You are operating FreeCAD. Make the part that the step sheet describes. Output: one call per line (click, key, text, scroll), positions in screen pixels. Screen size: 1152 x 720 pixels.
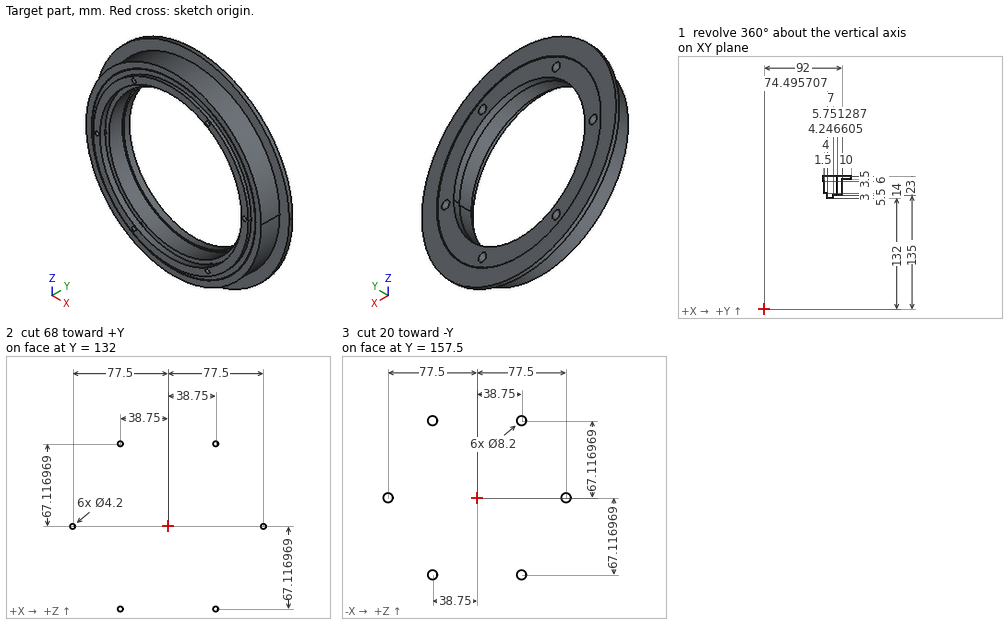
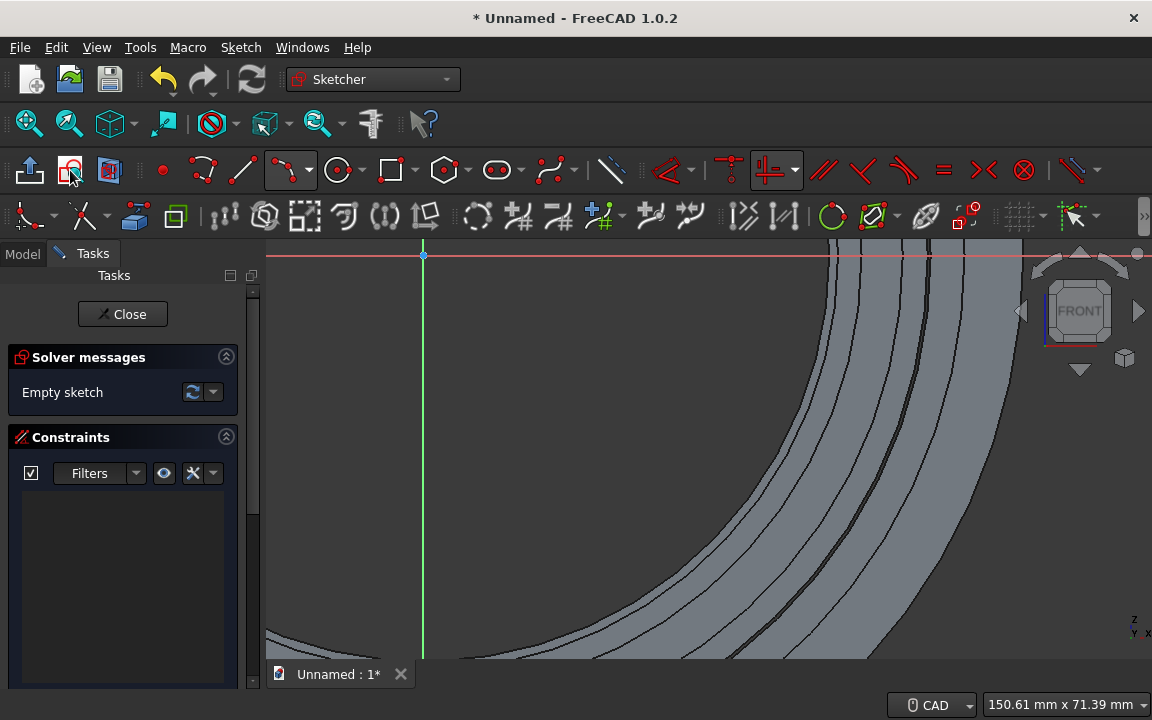
scroll(734, 532, down, 6)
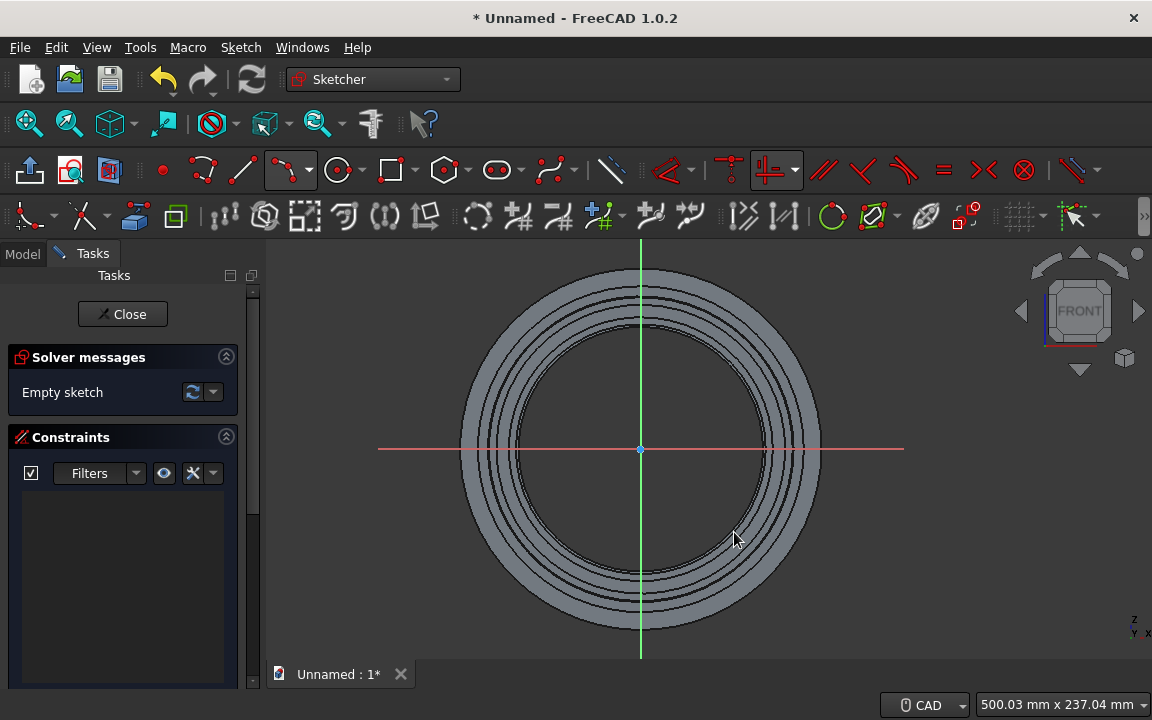
click(338, 170)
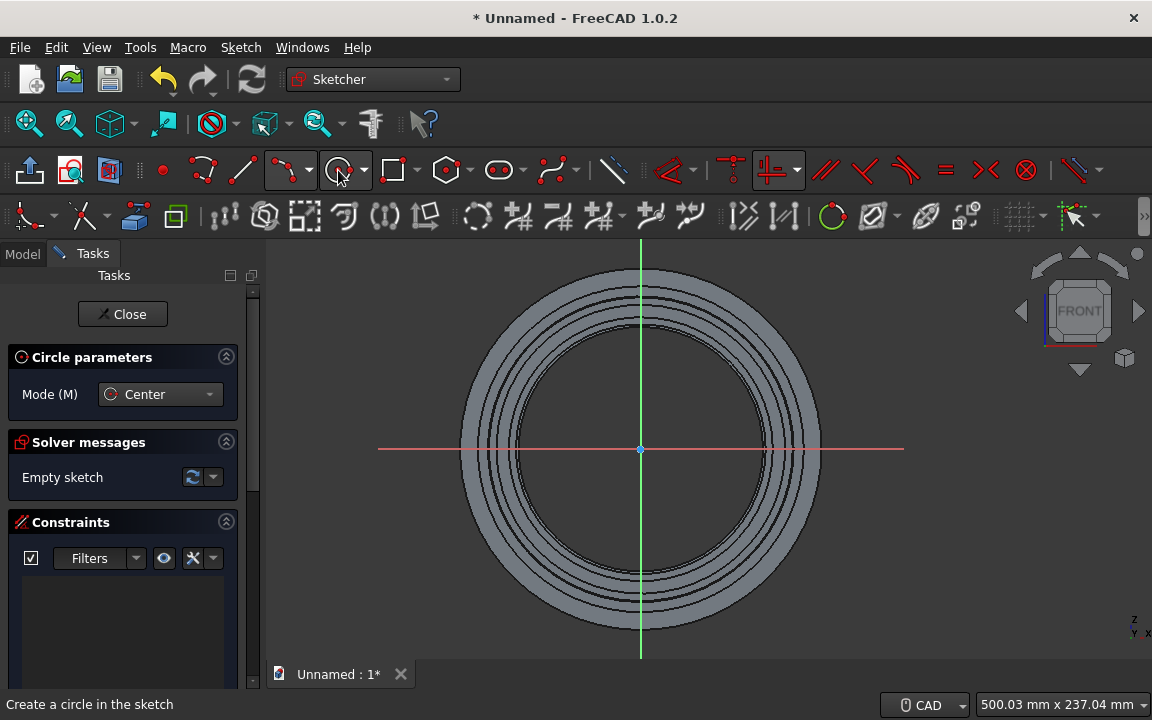
scroll(503, 449, up, 10)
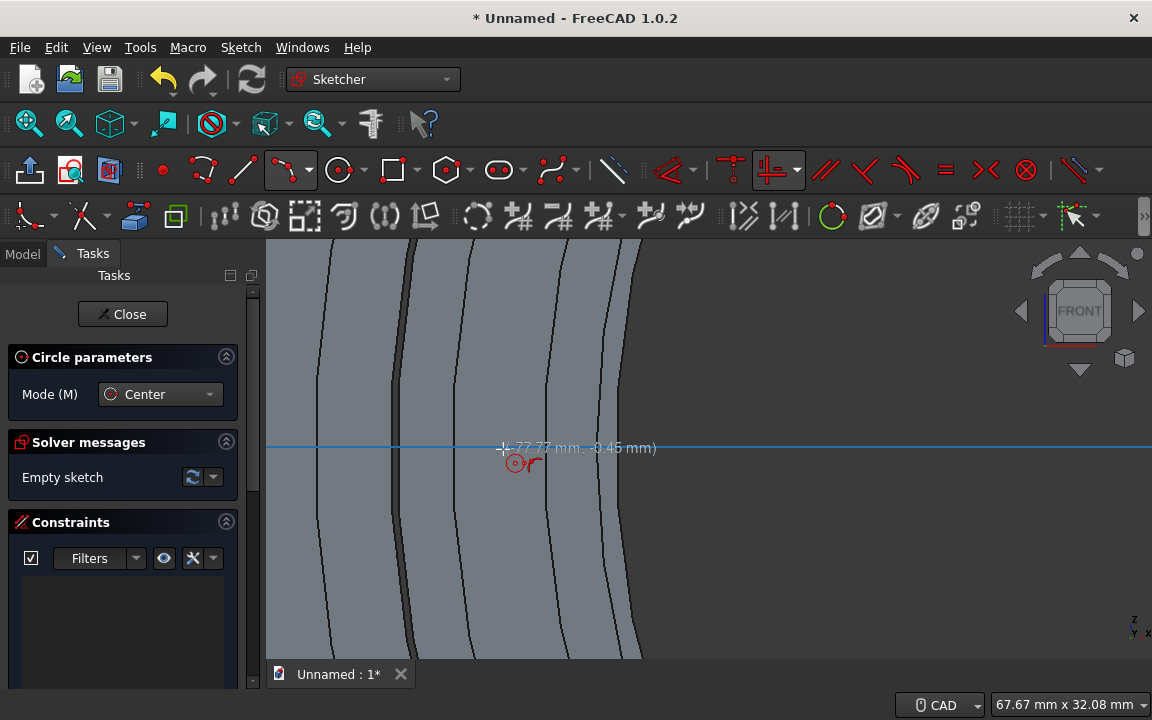
scroll(503, 449, down, 10)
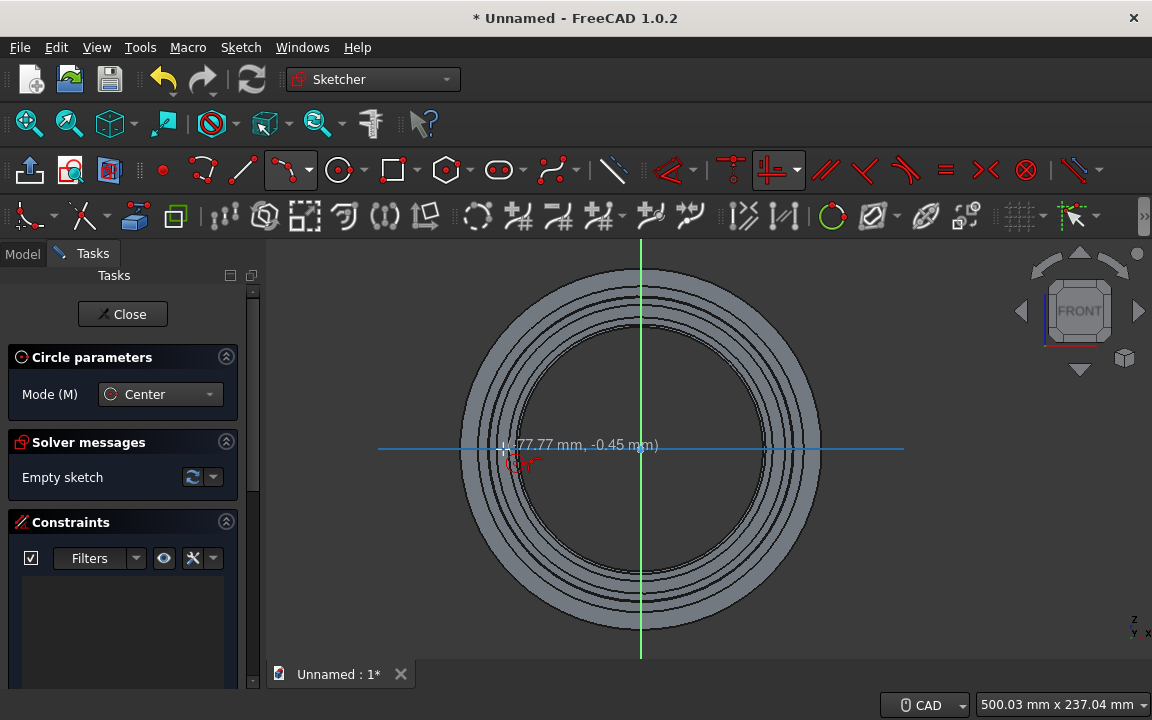
click(503, 449)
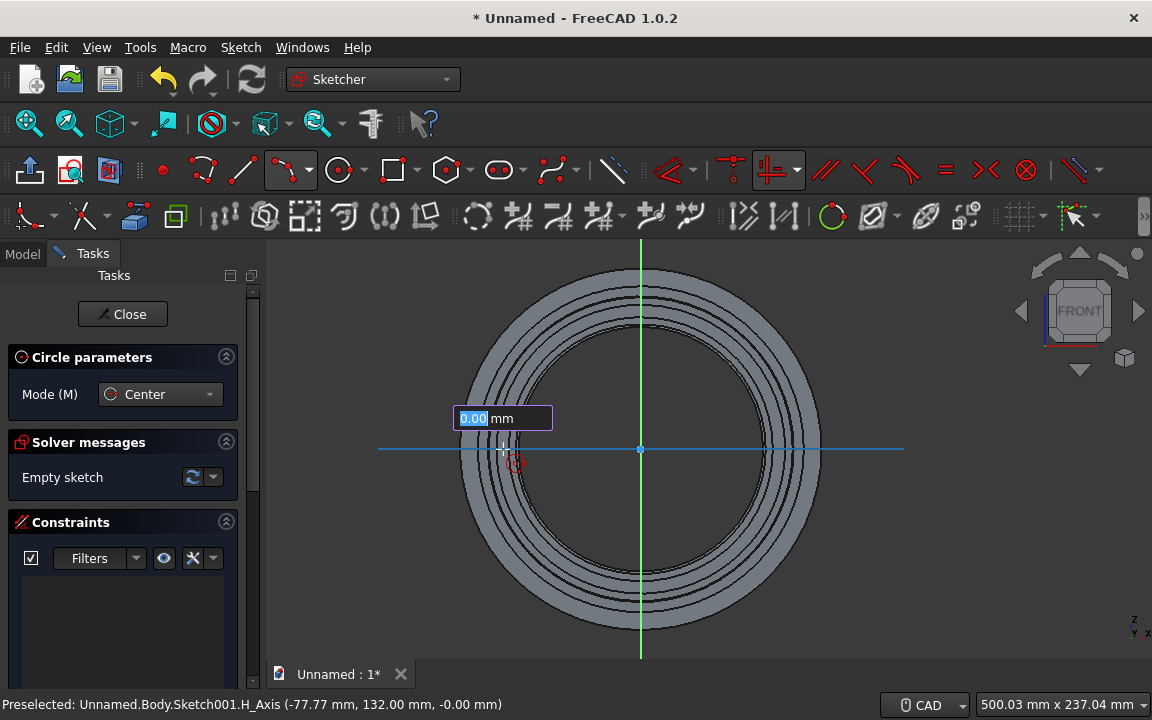
scroll(502, 453, up, 8)
move(502, 450)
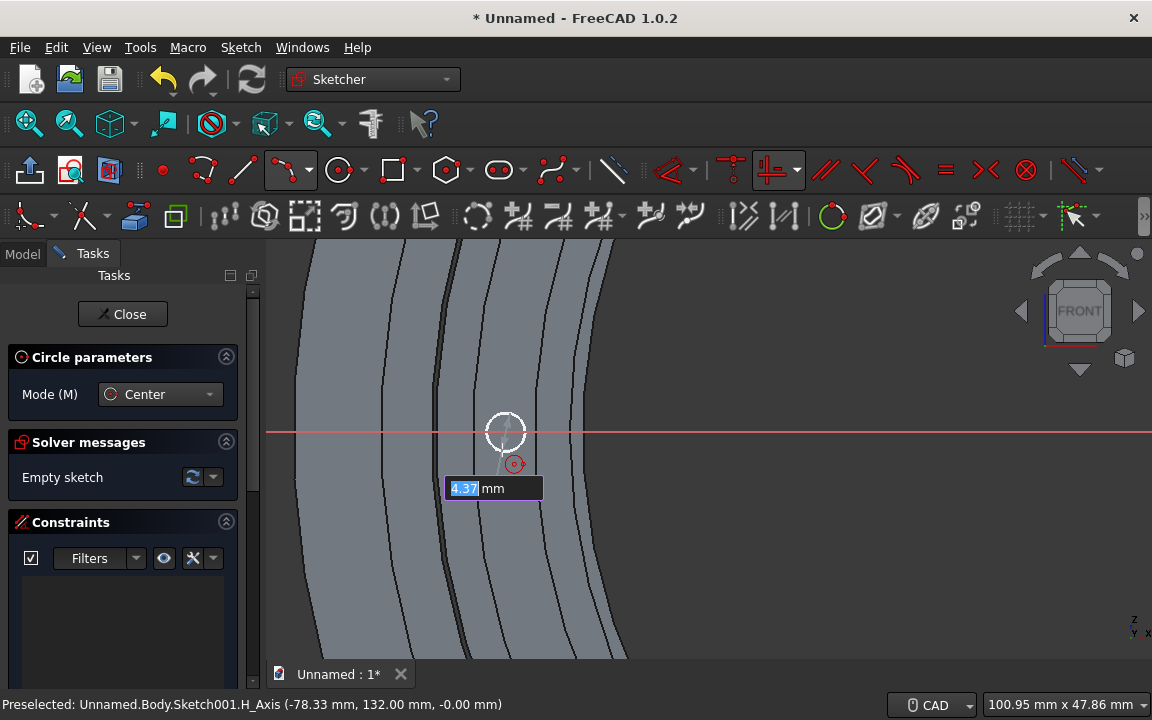
text(4.2)
key(Return)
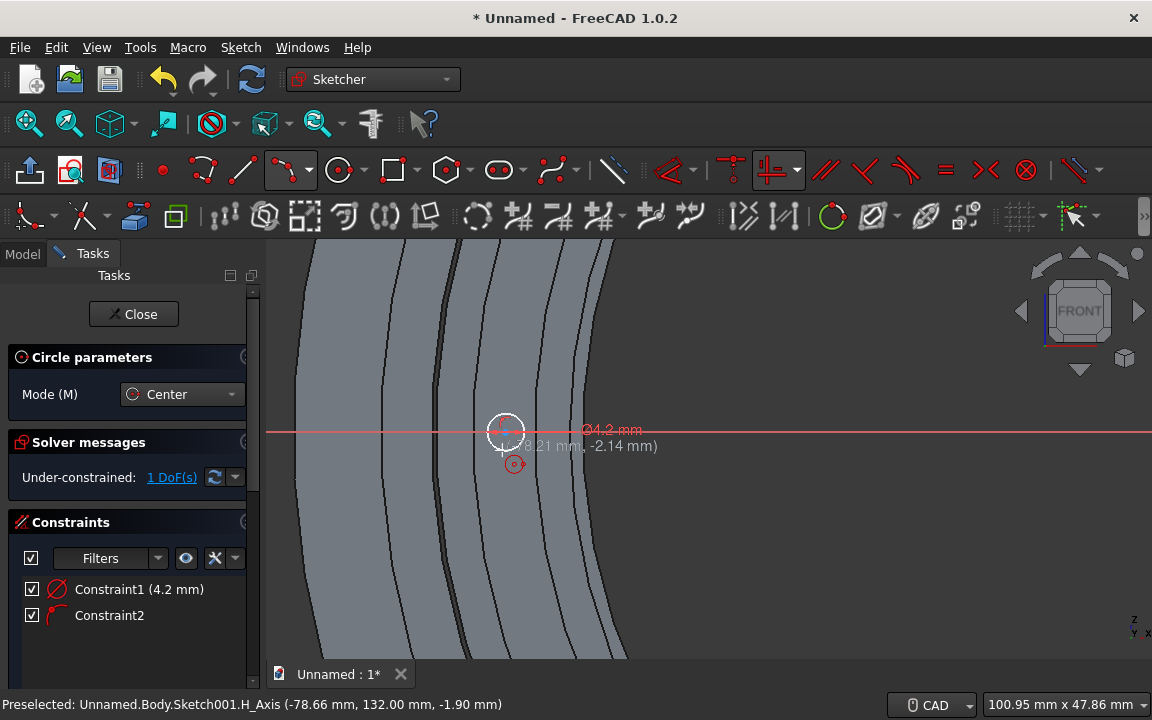
scroll(502, 453, down, 8)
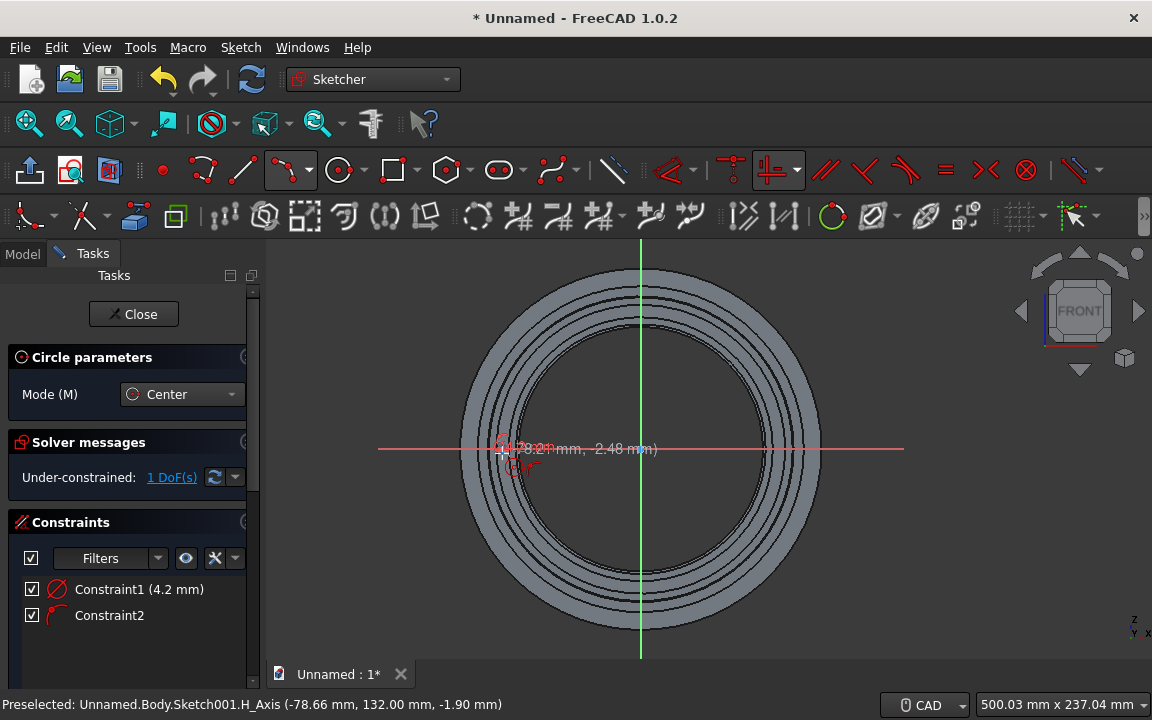
scroll(572, 330, up, 10)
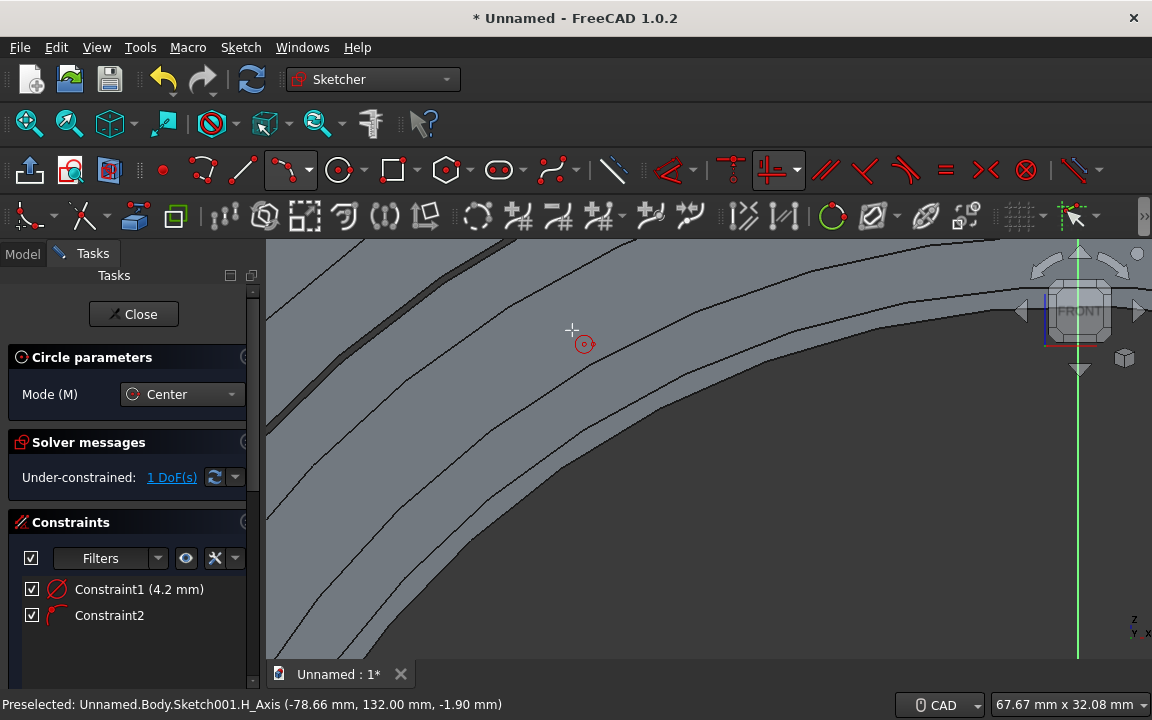
scroll(572, 330, down, 10)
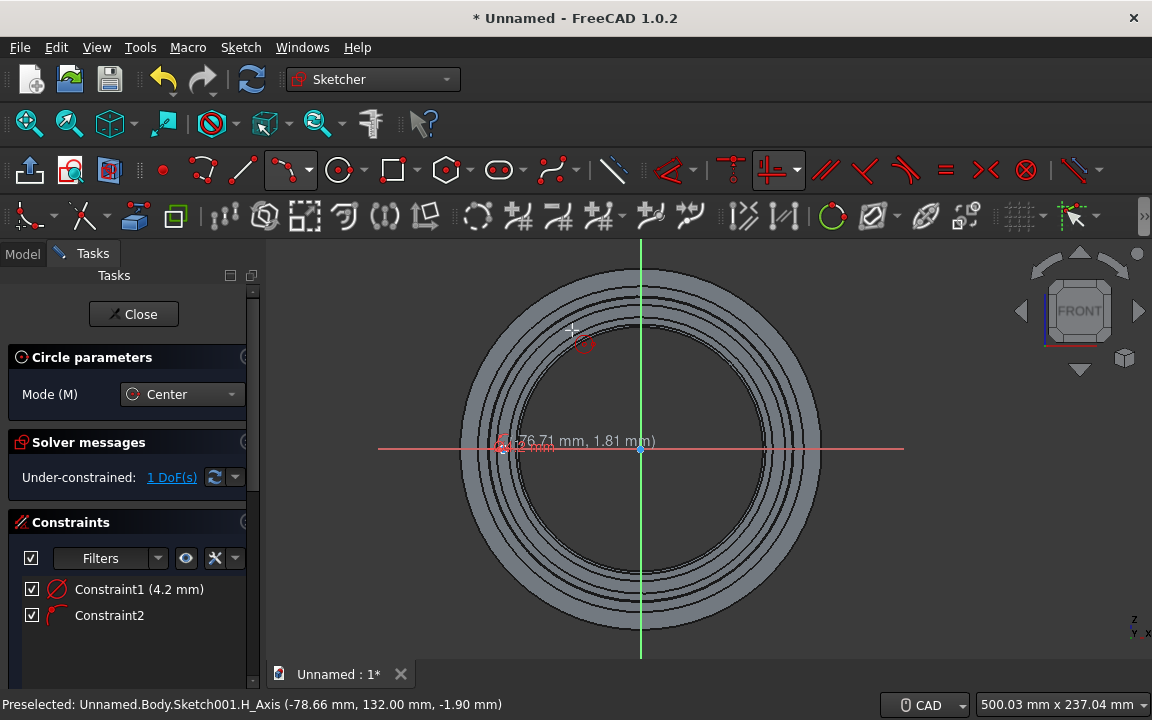
click(572, 330)
move(575, 328)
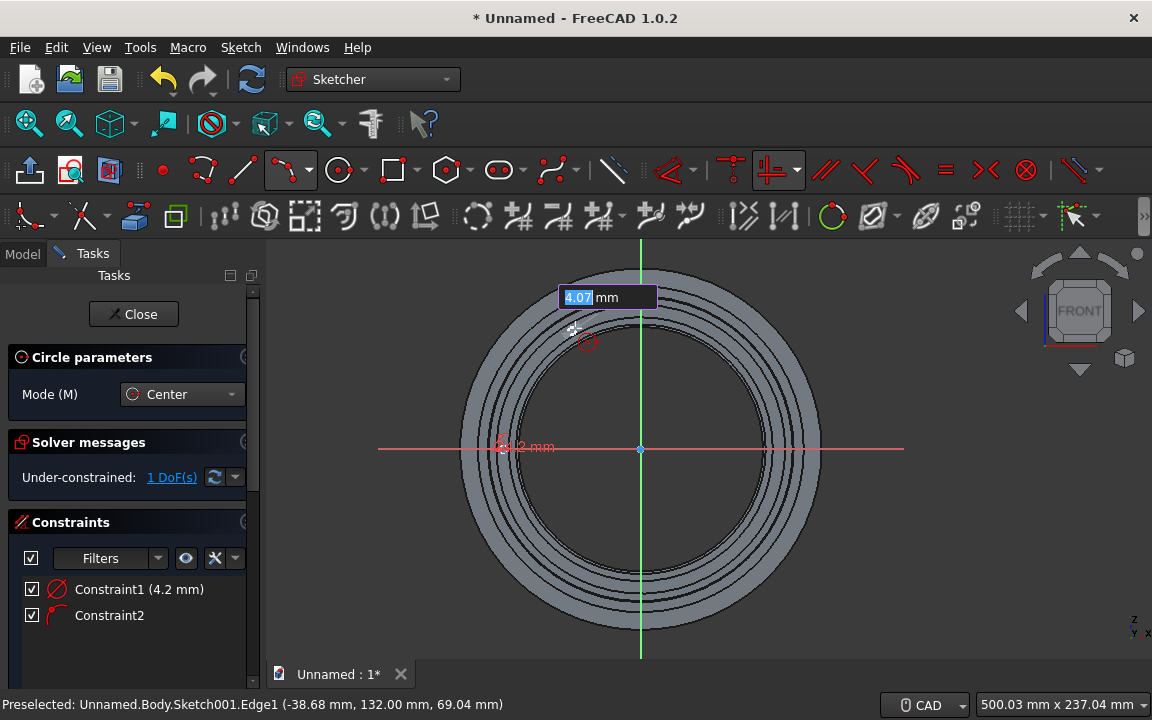
text(4.2)
key(Return)